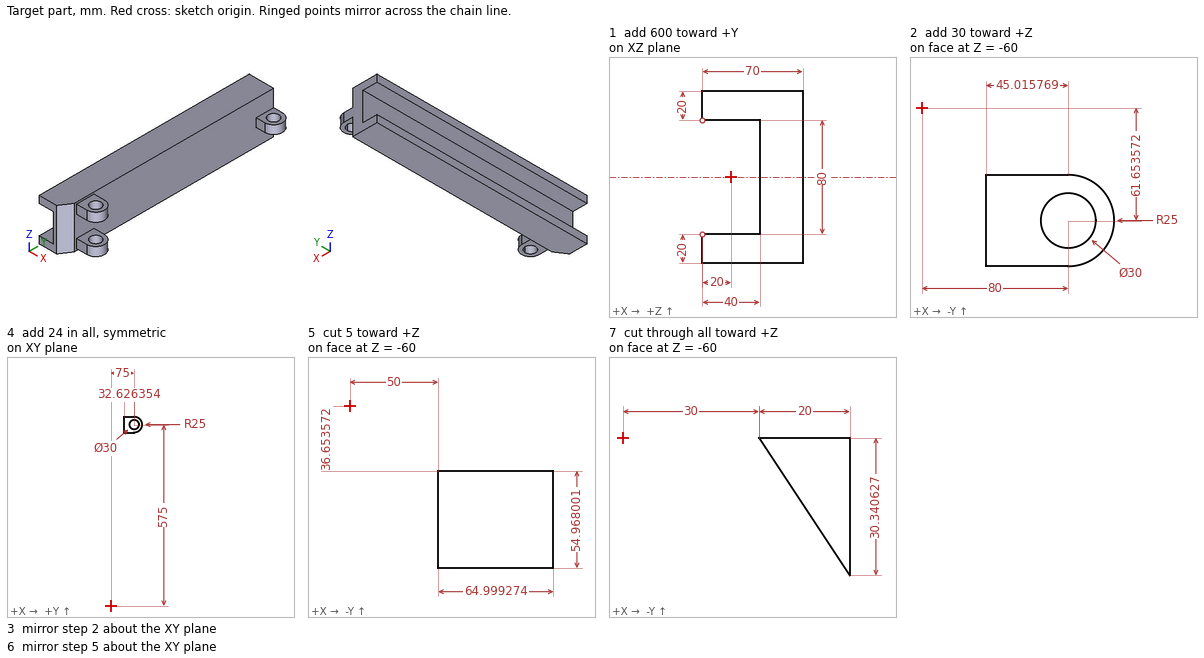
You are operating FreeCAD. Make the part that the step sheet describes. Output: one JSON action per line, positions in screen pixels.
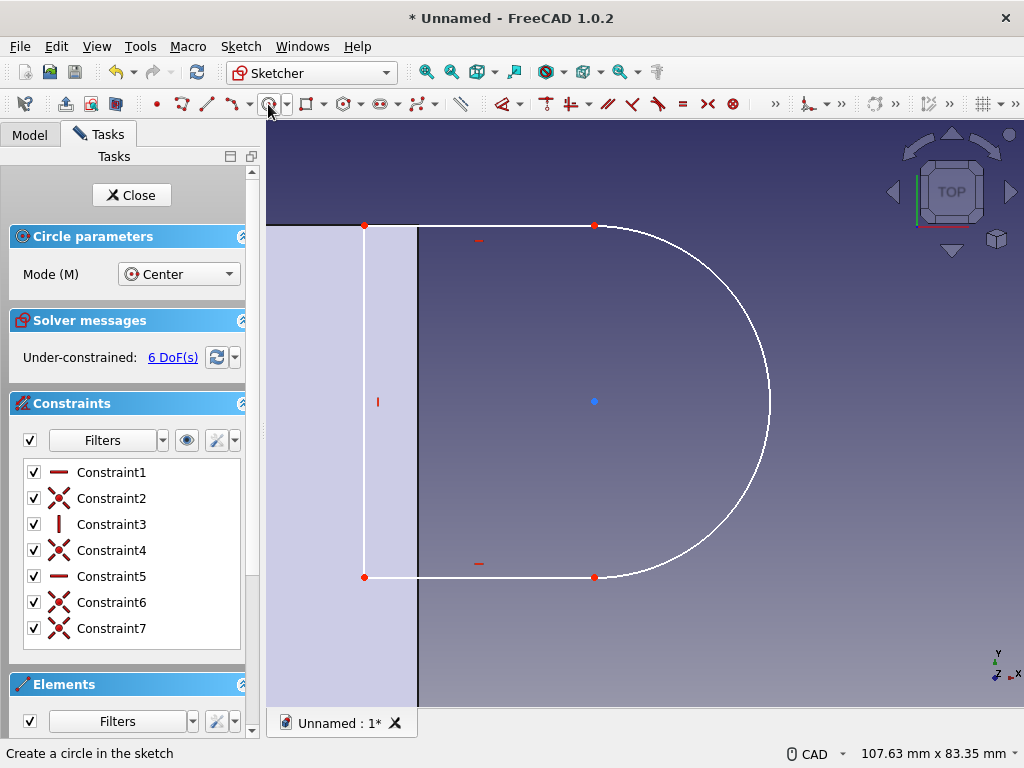
{"action": "left_click", "coordinate": [594, 401]}
{"action": "mouse_move", "coordinate": [669, 327]}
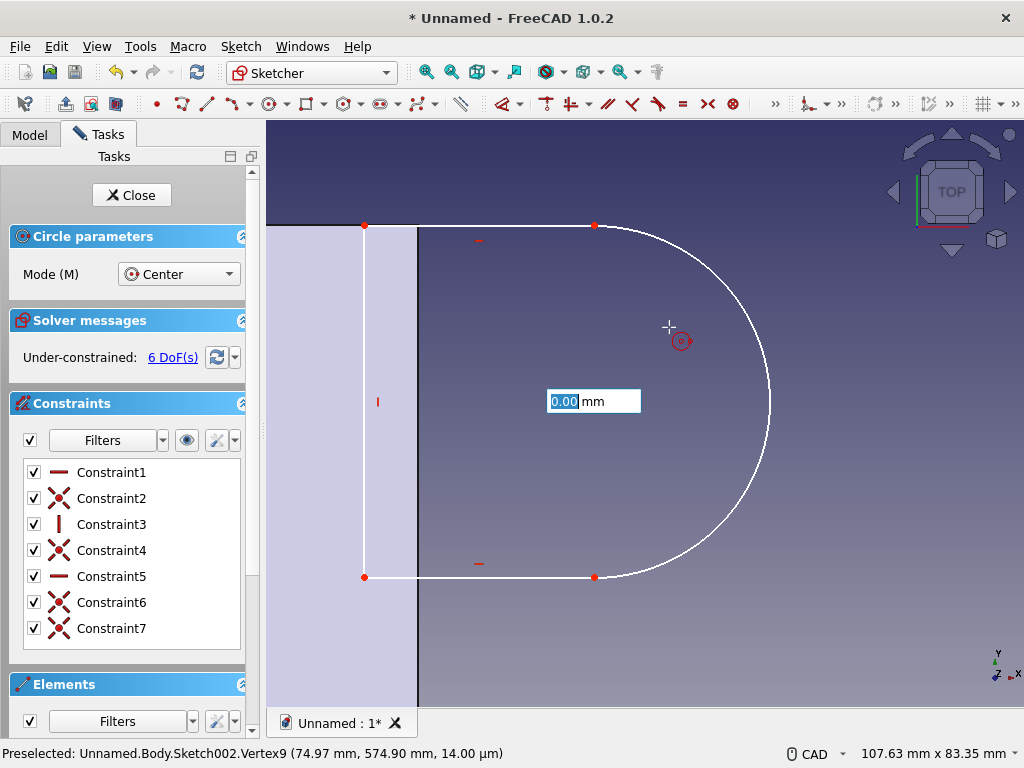
{"action": "type", "text": "30"}
{"action": "key", "text": "Return"}
{"action": "key", "text": "Escape"}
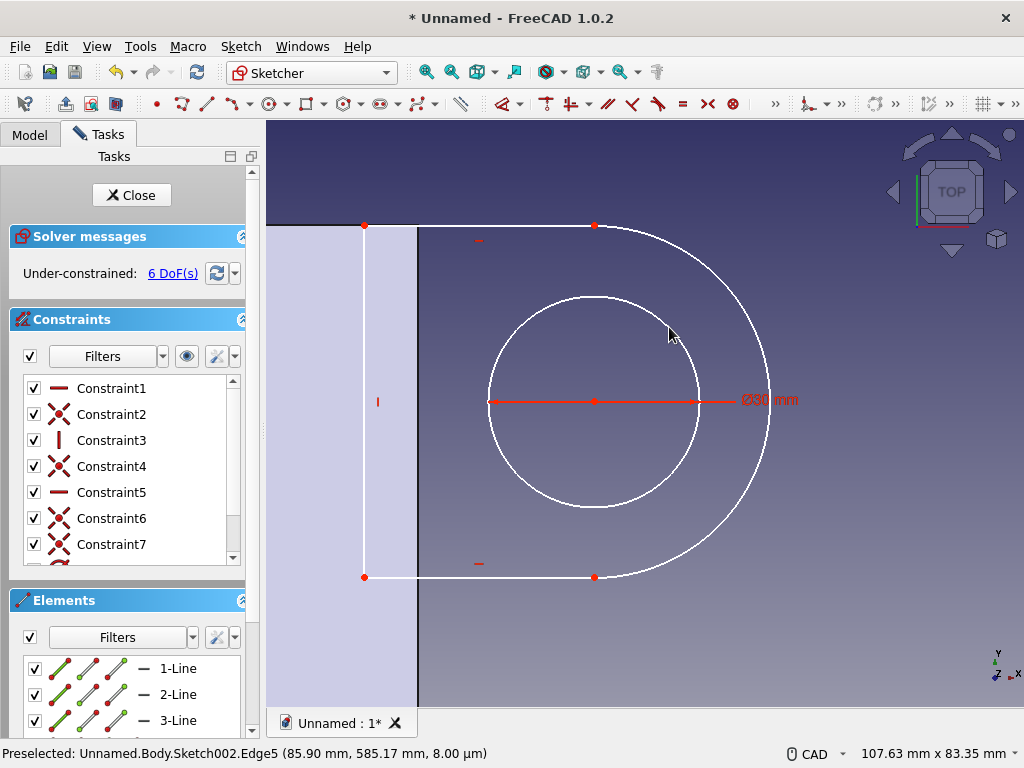
{"action": "left_click", "coordinate": [525, 226]}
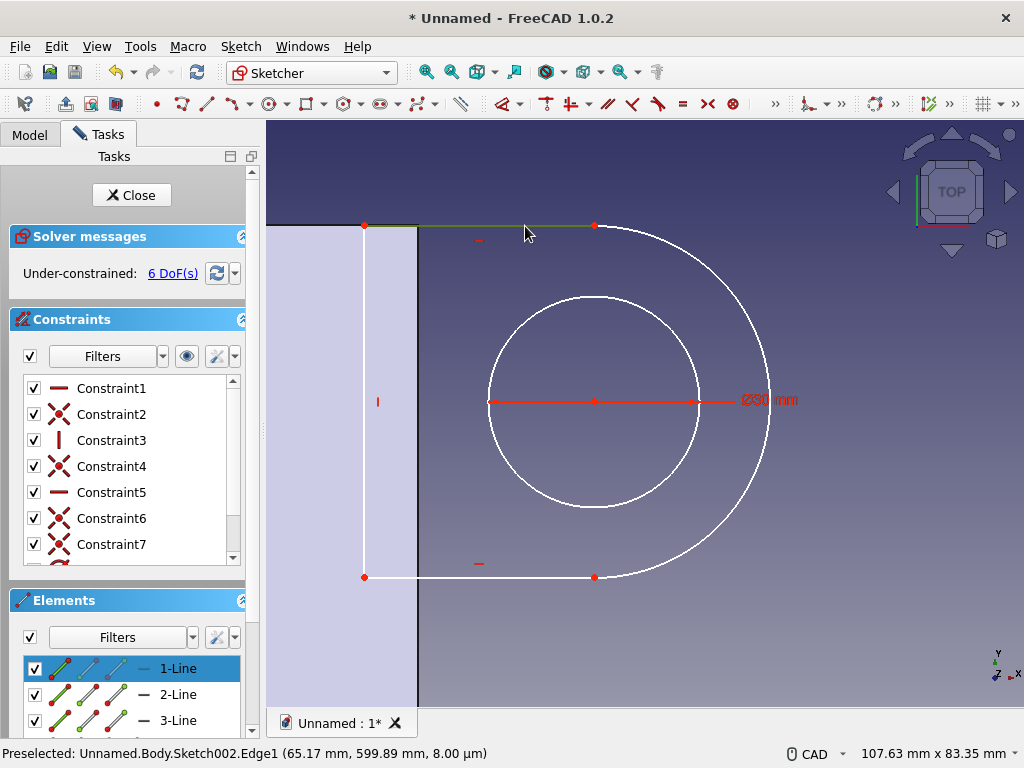
{"action": "left_click", "coordinate": [736, 505]}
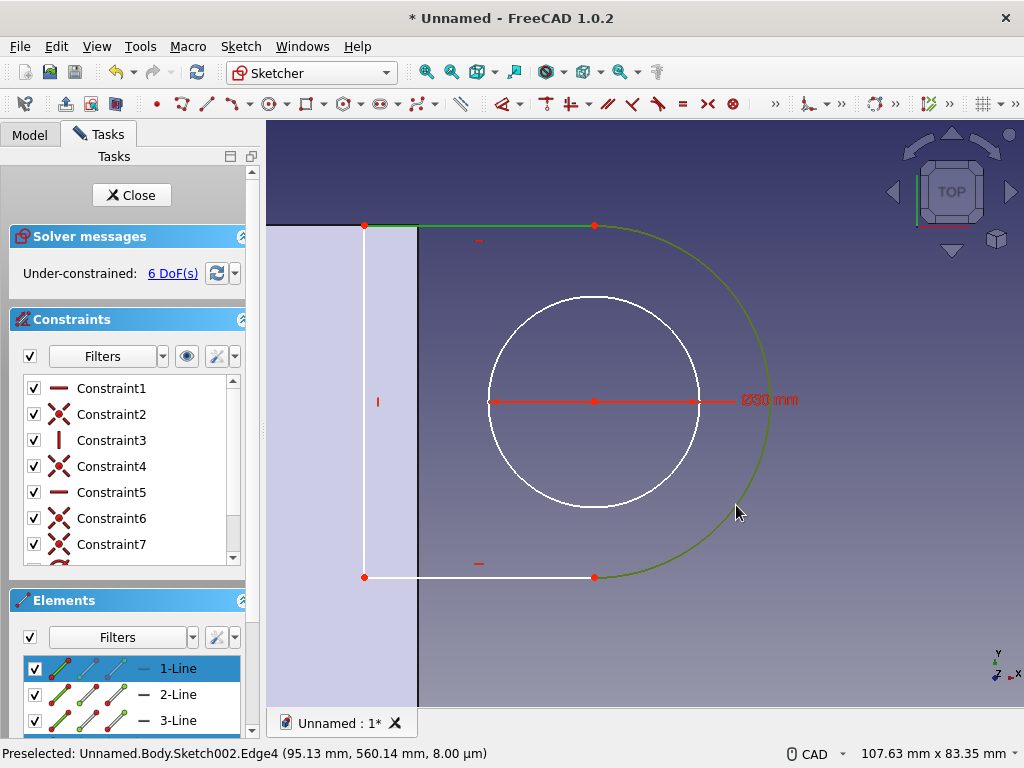
{"action": "left_click", "coordinate": [658, 104]}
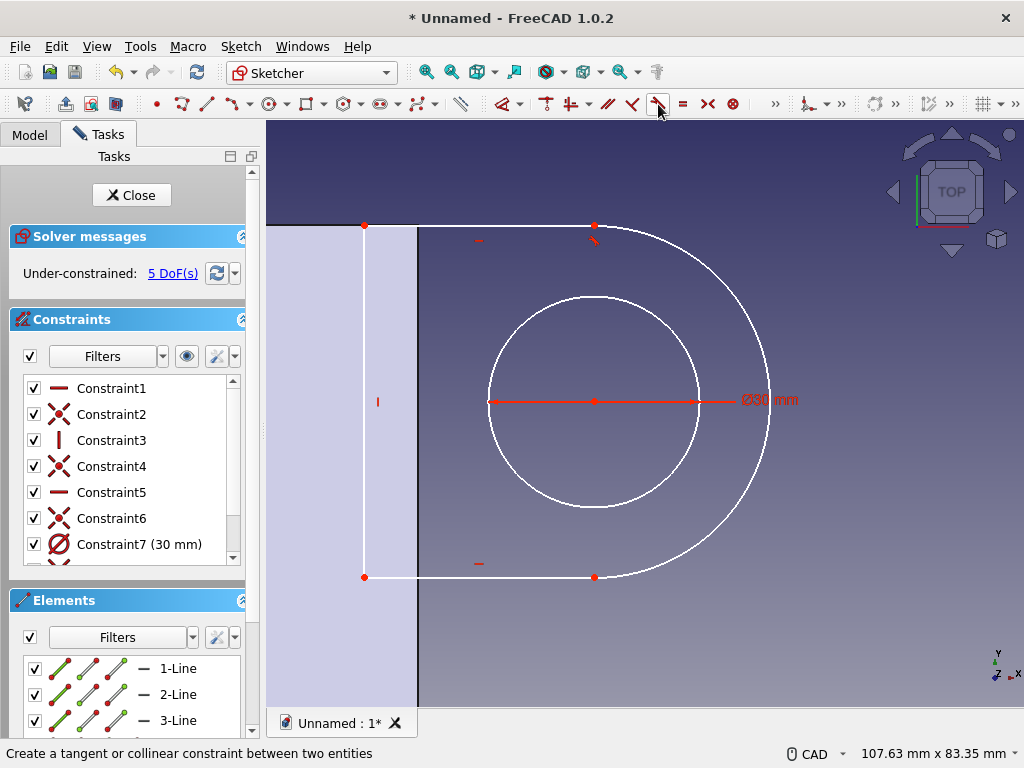
{"action": "left_click", "coordinate": [433, 578]}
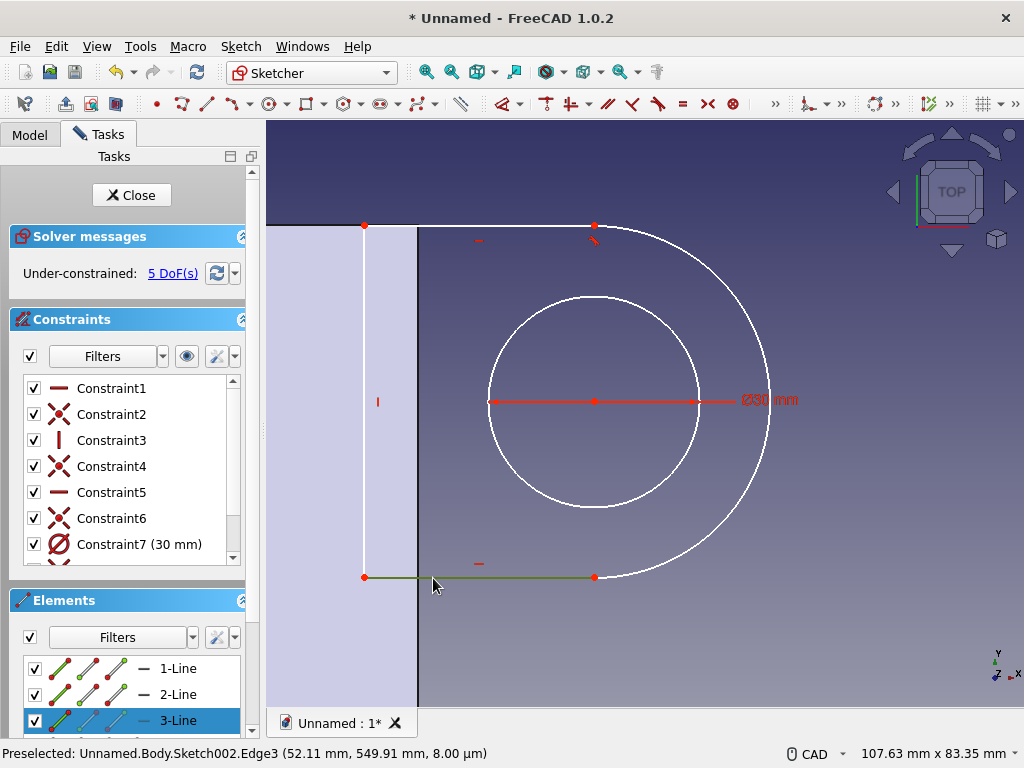
{"action": "left_click", "coordinate": [736, 505]}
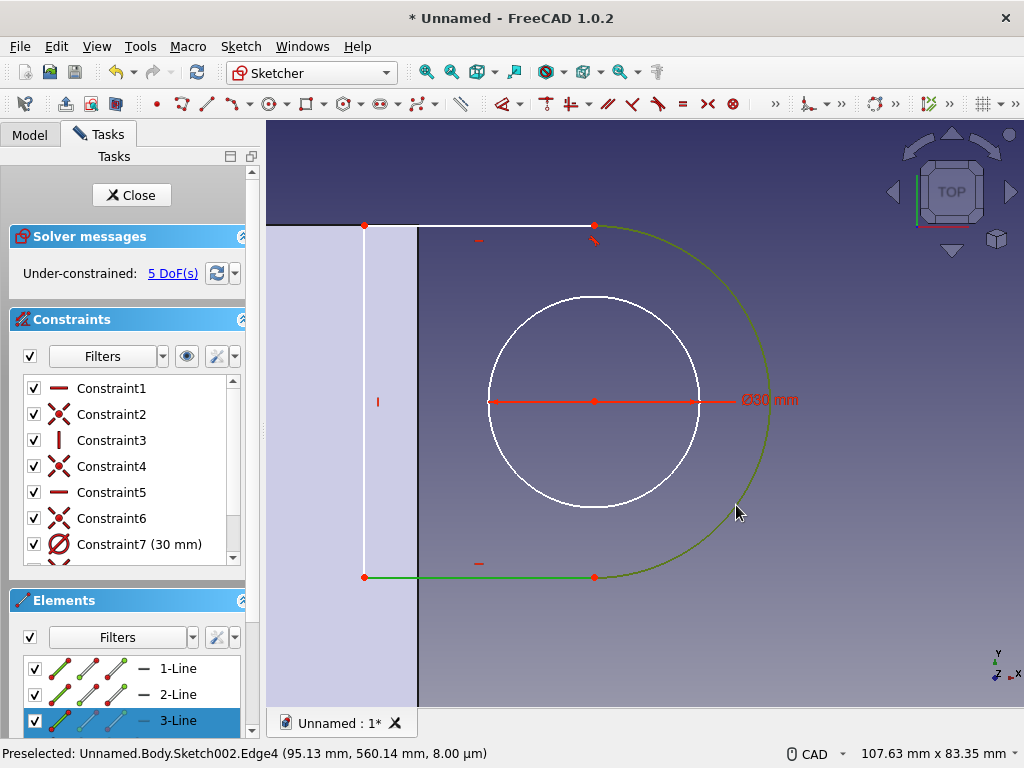
{"action": "left_click", "coordinate": [658, 104]}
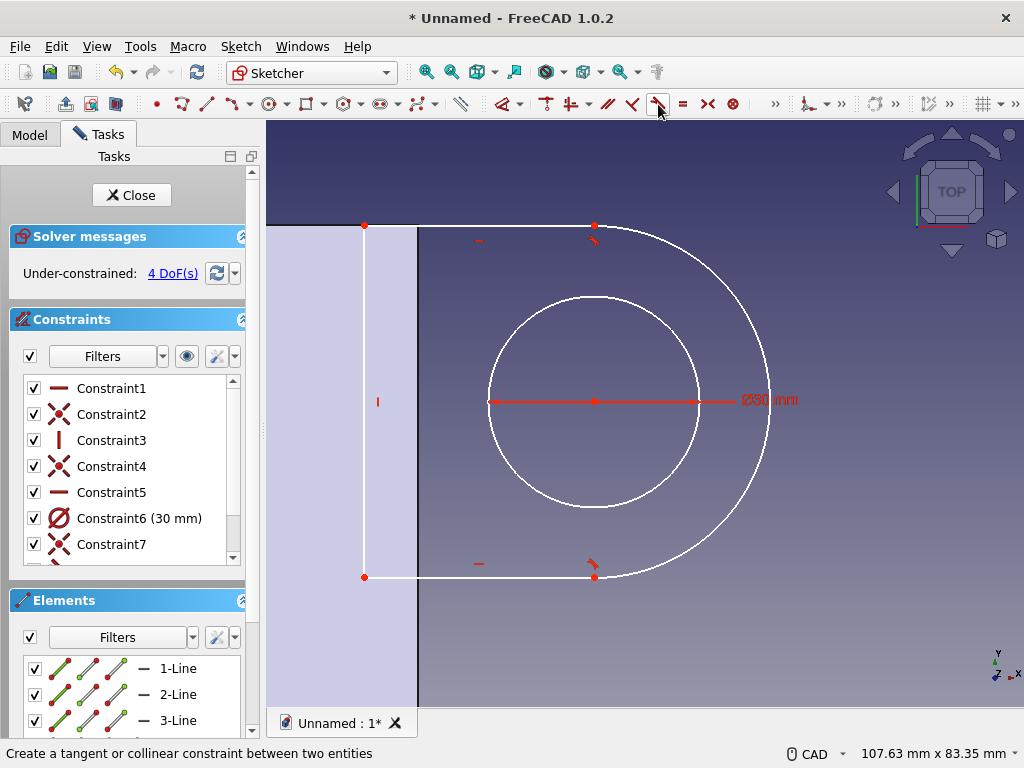
{"action": "left_click", "coordinate": [502, 104]}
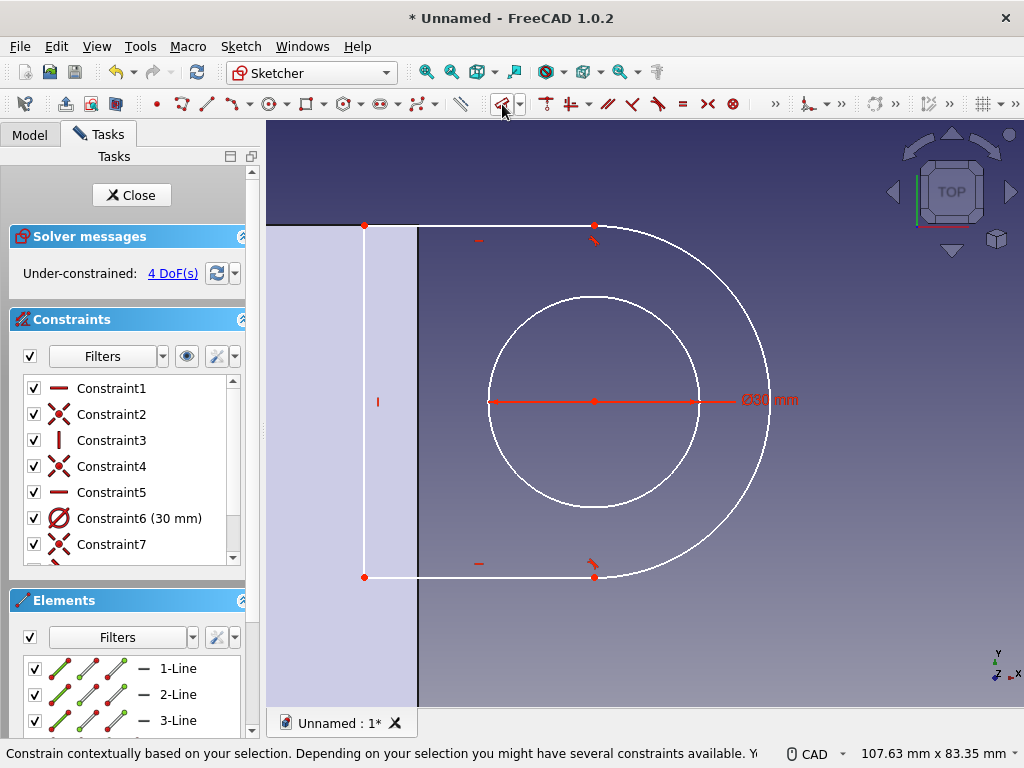
{"action": "left_click", "coordinate": [736, 505]}
{"action": "left_click", "coordinate": [762, 524]}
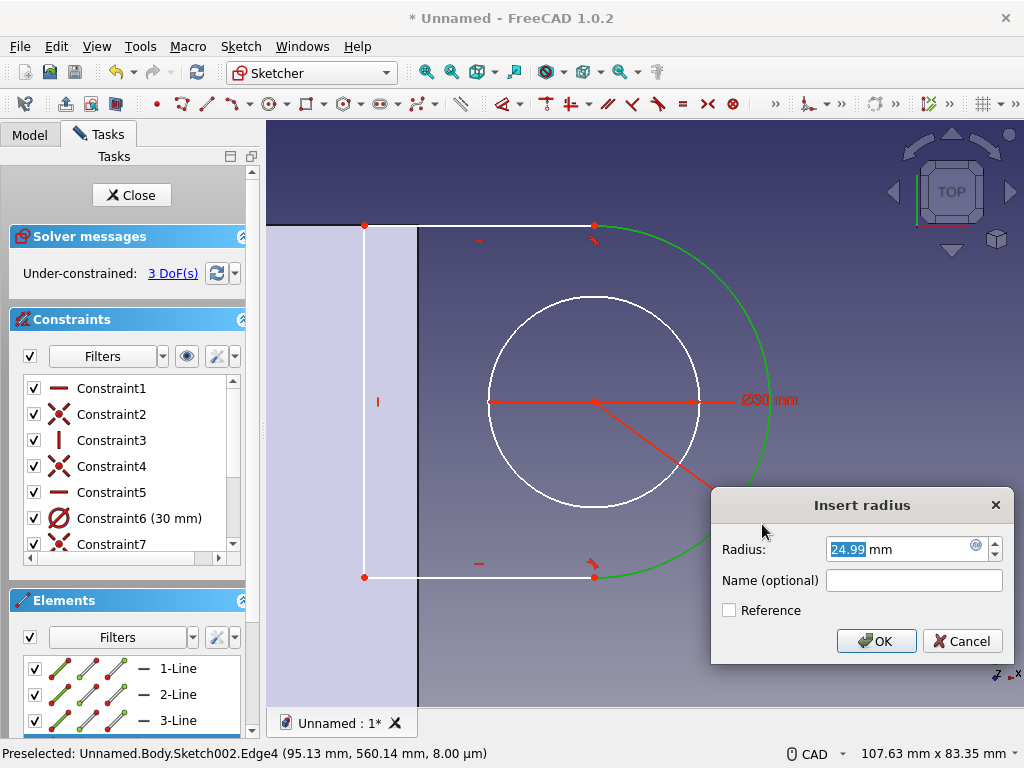
{"action": "type", "text": "25"}
{"action": "key", "text": "Return"}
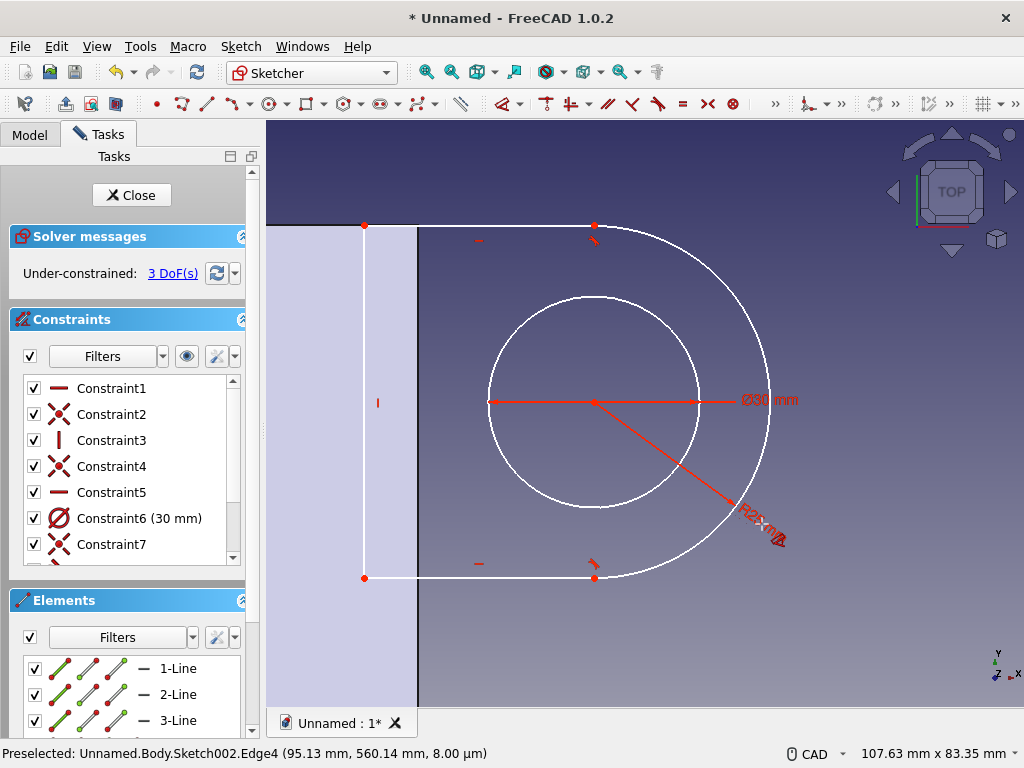
{"action": "left_click", "coordinate": [594, 402]}
{"action": "left_click", "coordinate": [444, 368]}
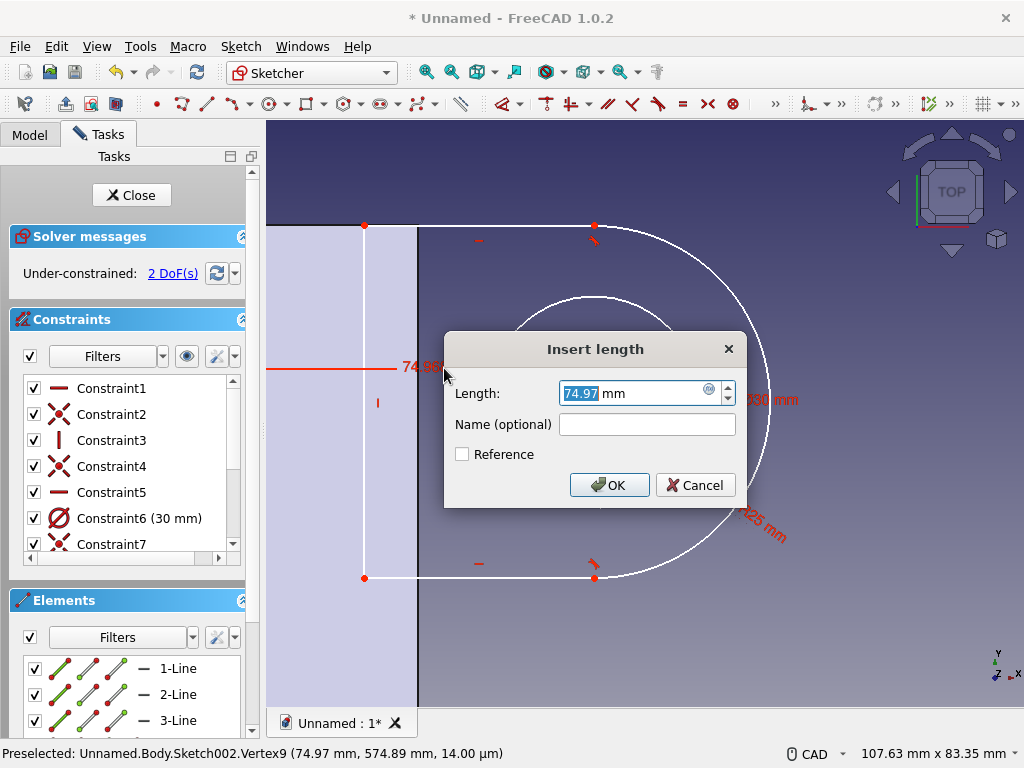
{"action": "type", "text": "75"}
{"action": "key", "text": "Return"}